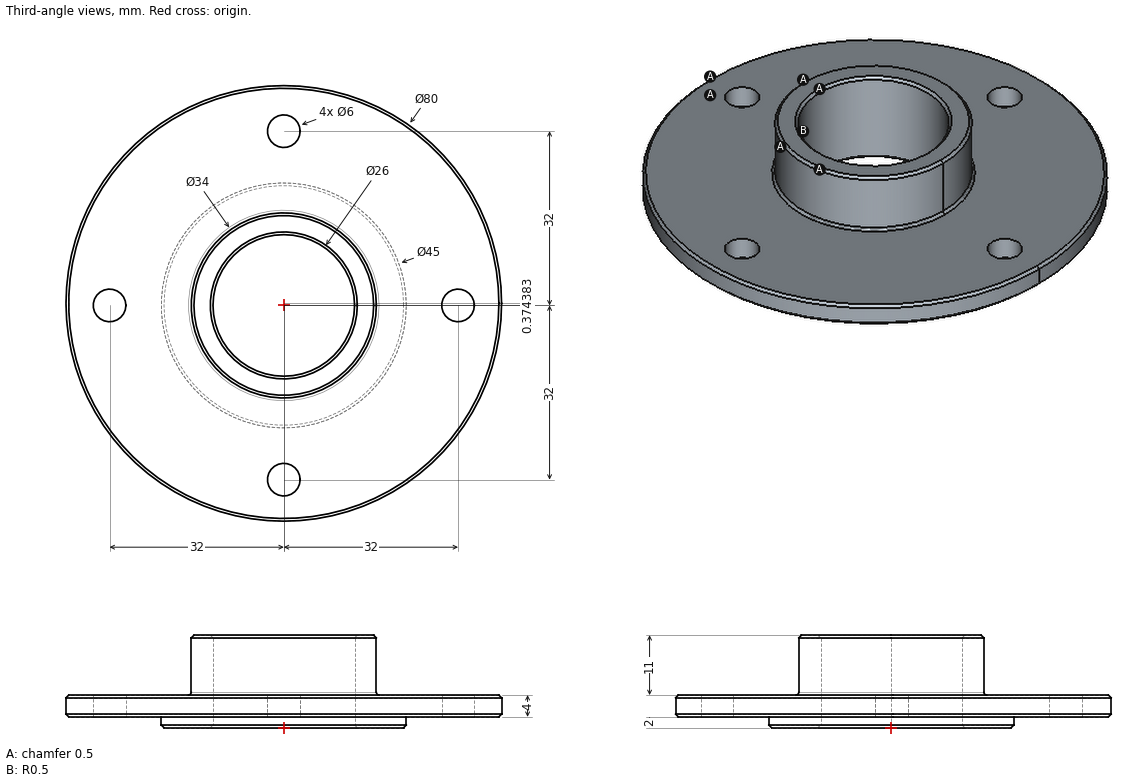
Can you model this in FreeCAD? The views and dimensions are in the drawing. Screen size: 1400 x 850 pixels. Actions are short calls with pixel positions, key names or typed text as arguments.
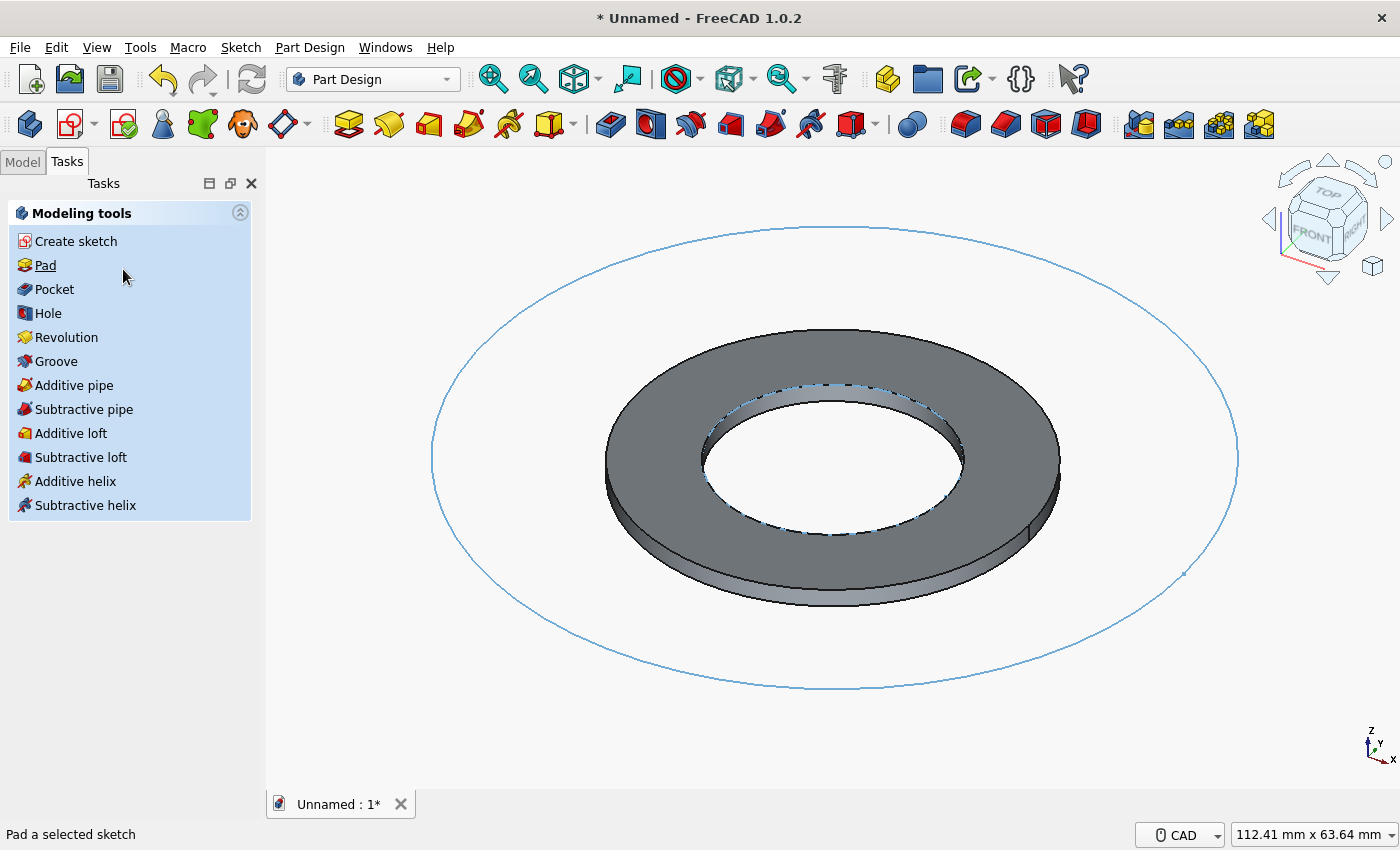
click(350, 124)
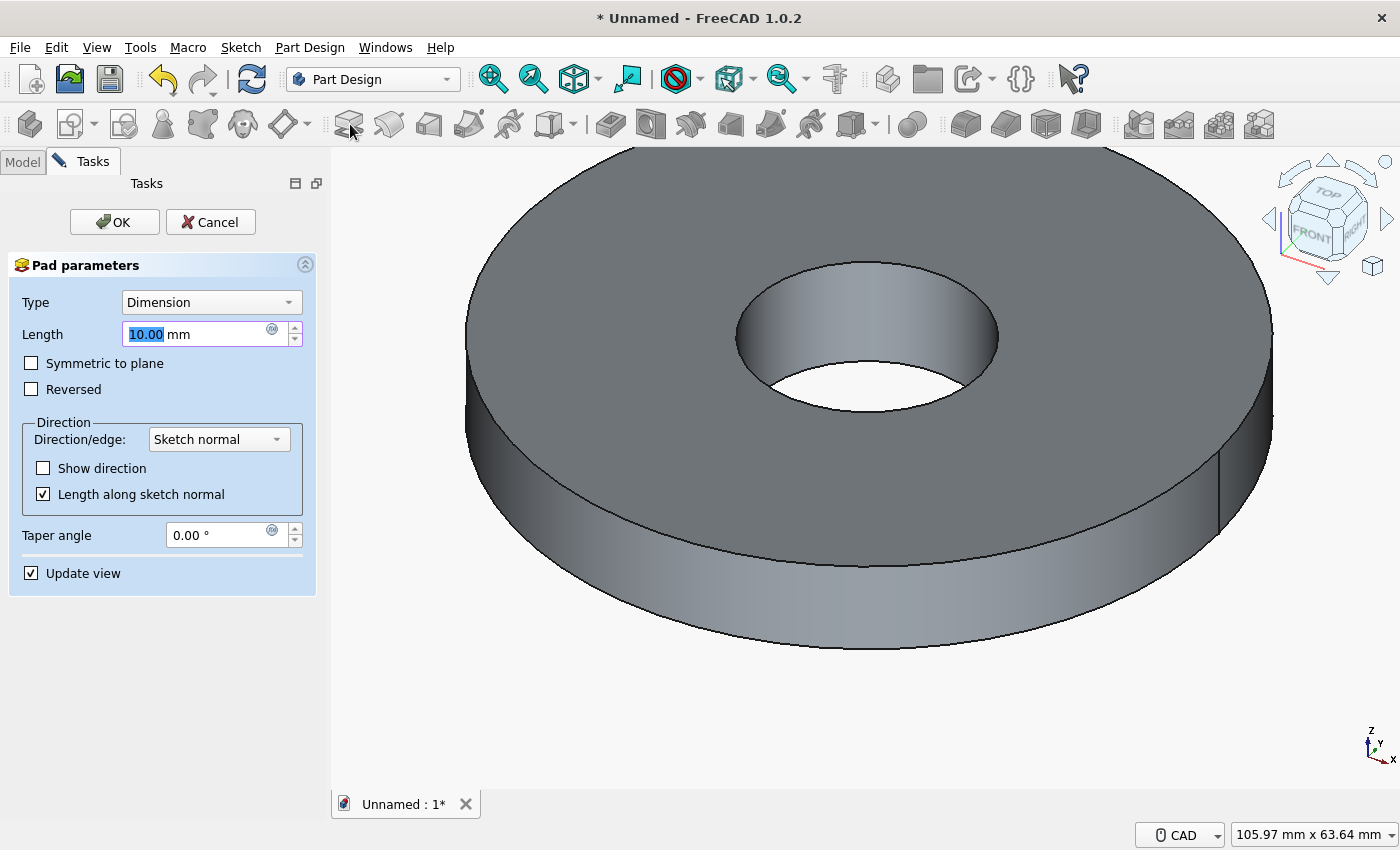
text(4)
key(Tab)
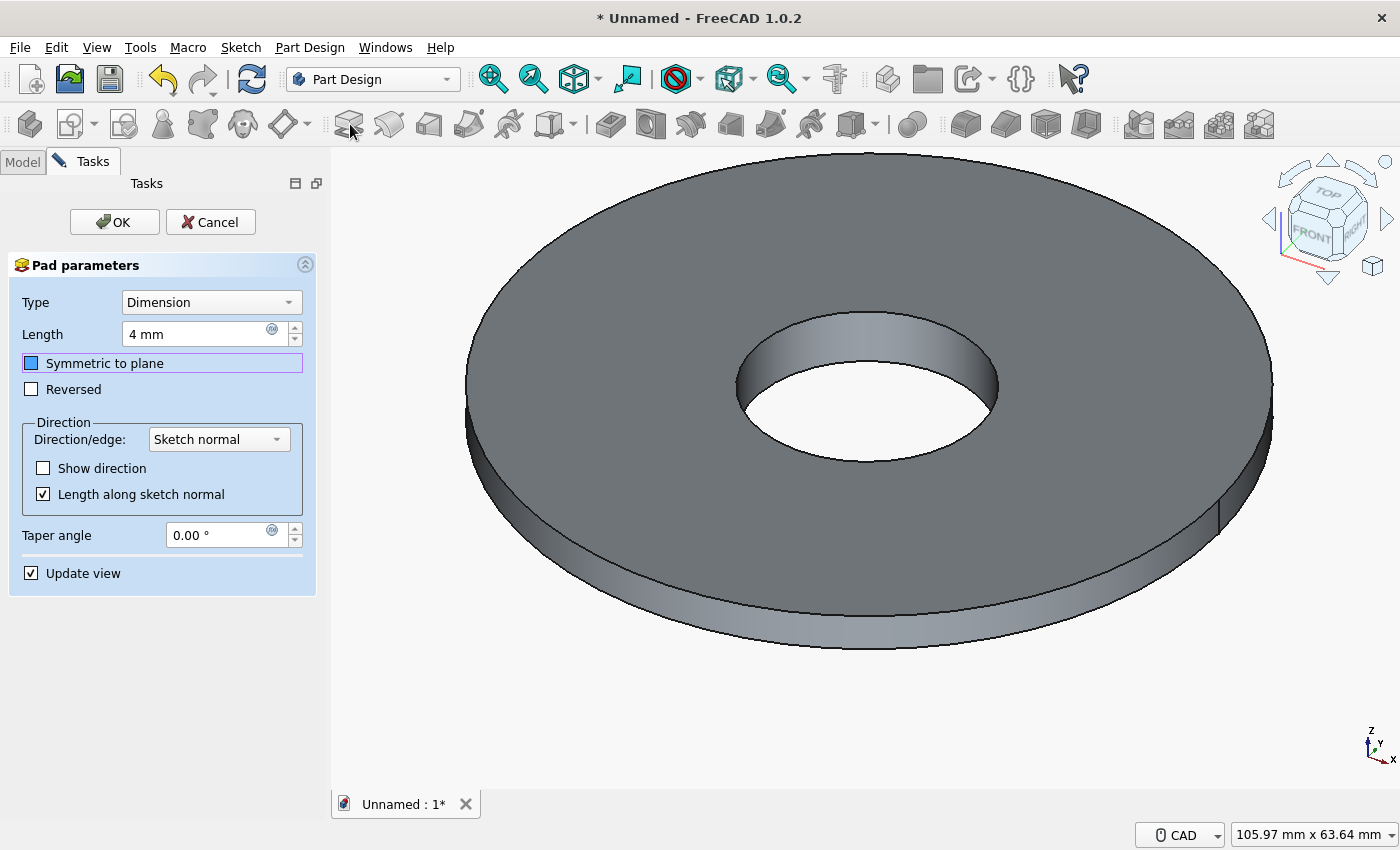
click(115, 222)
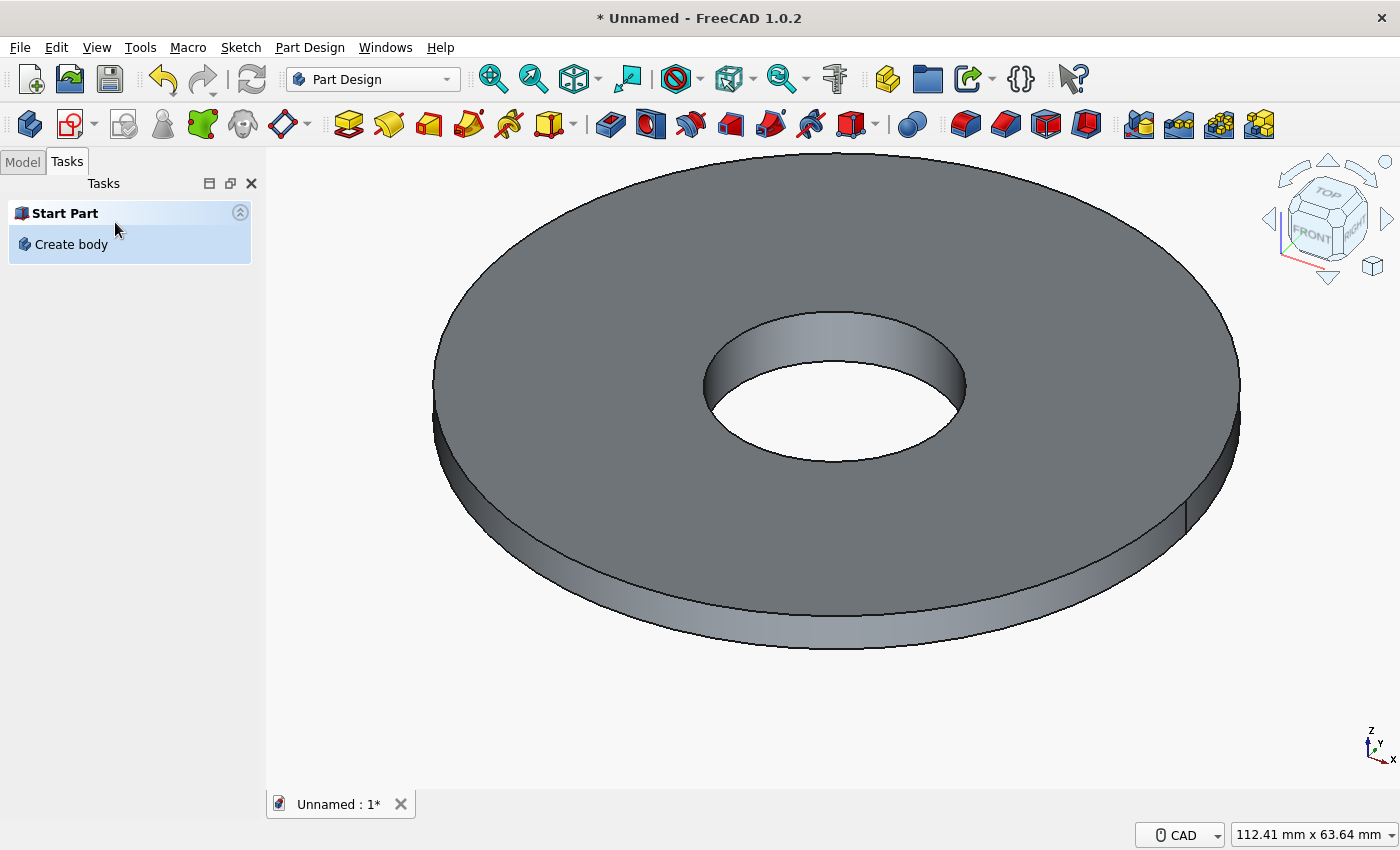
click(494, 80)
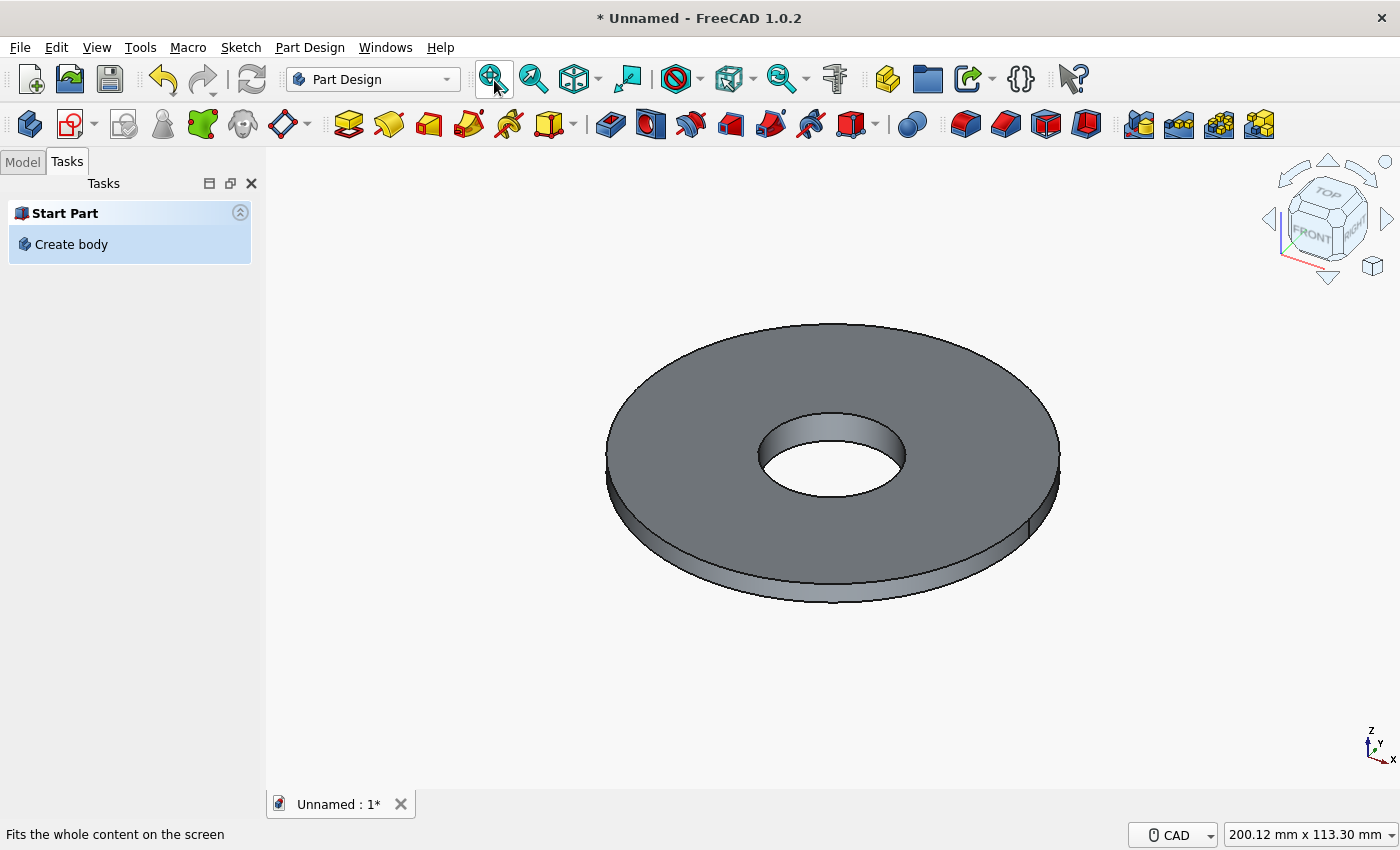
click(954, 407)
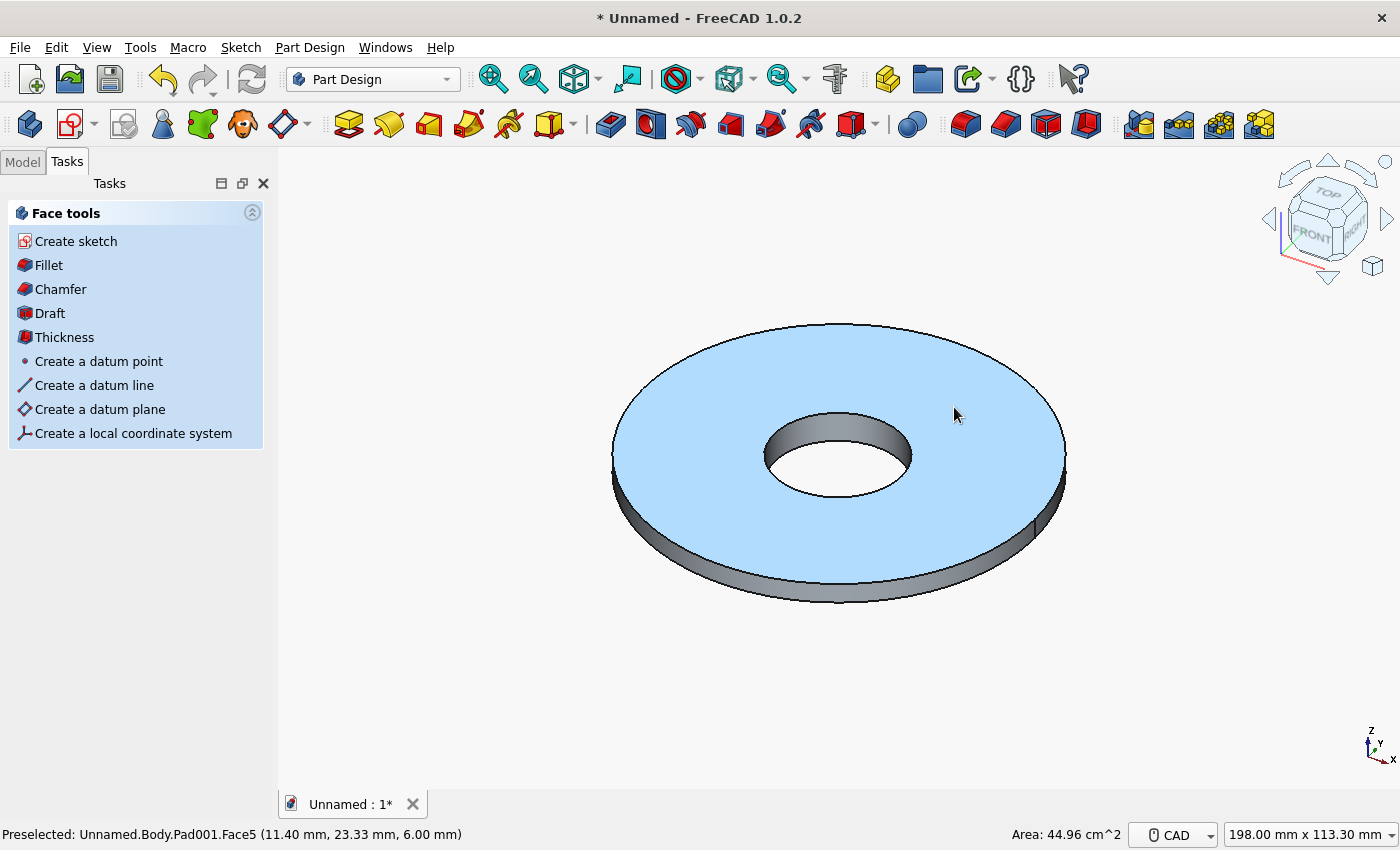
click(70, 124)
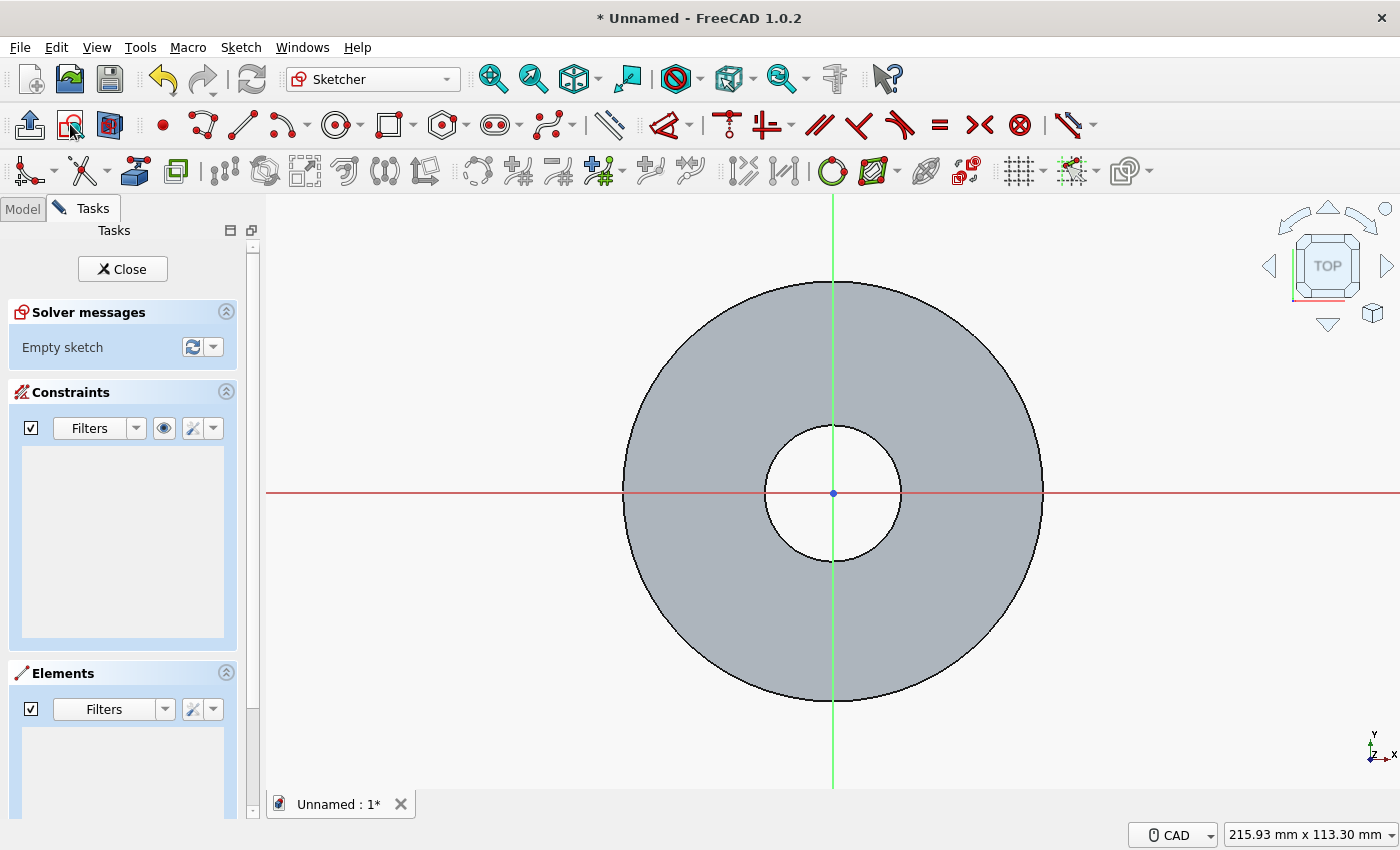
scroll(889, 495, up, 4)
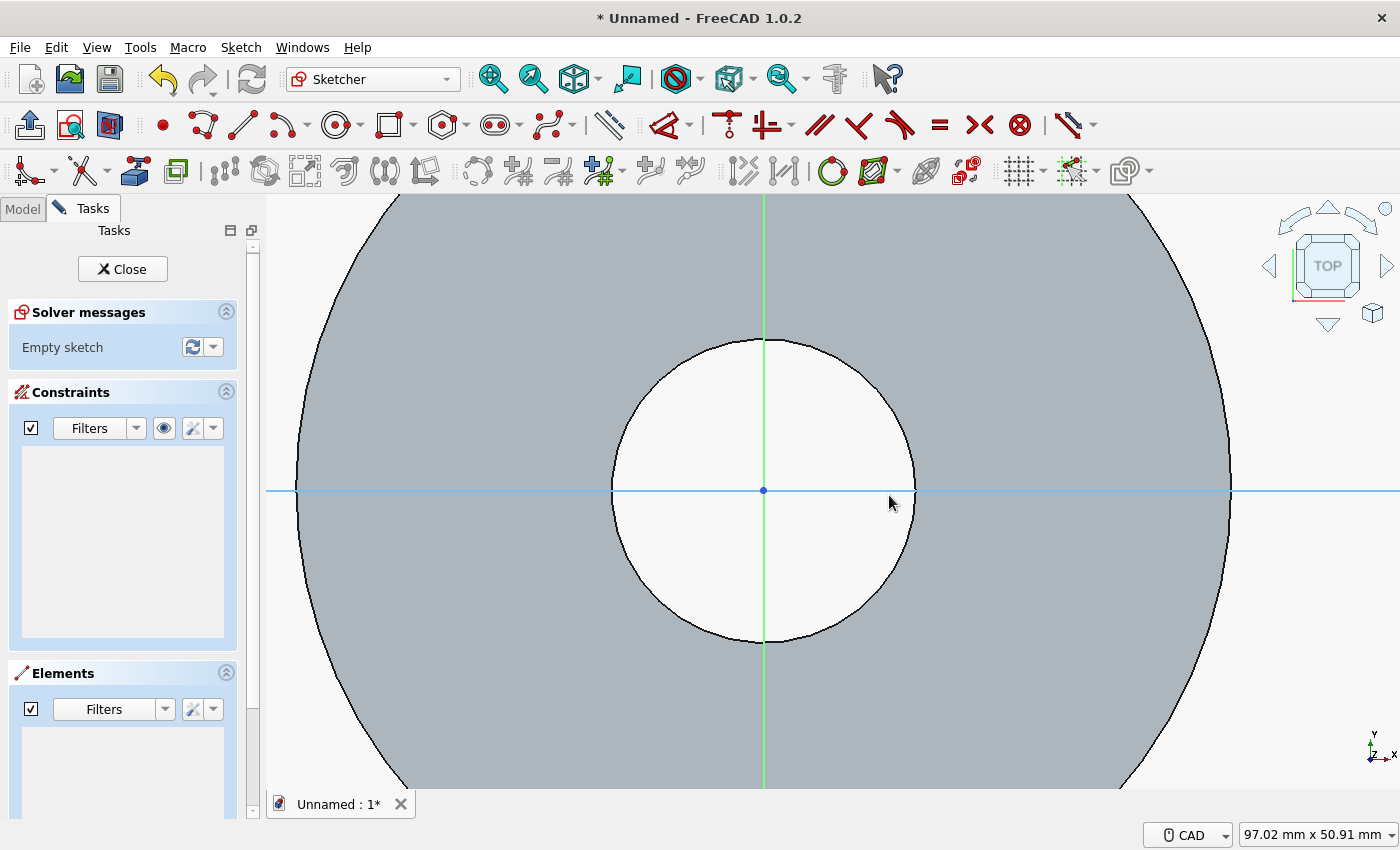
click(336, 126)